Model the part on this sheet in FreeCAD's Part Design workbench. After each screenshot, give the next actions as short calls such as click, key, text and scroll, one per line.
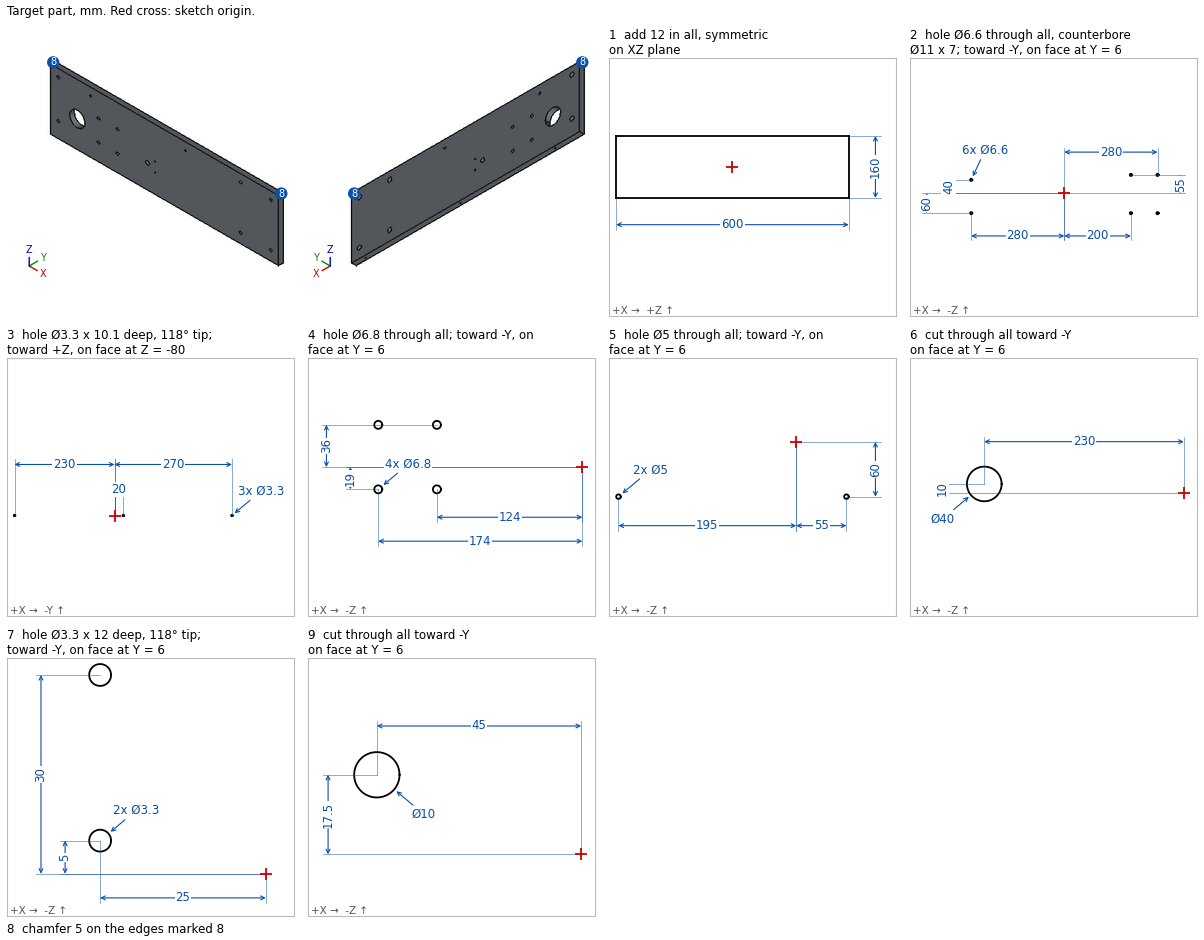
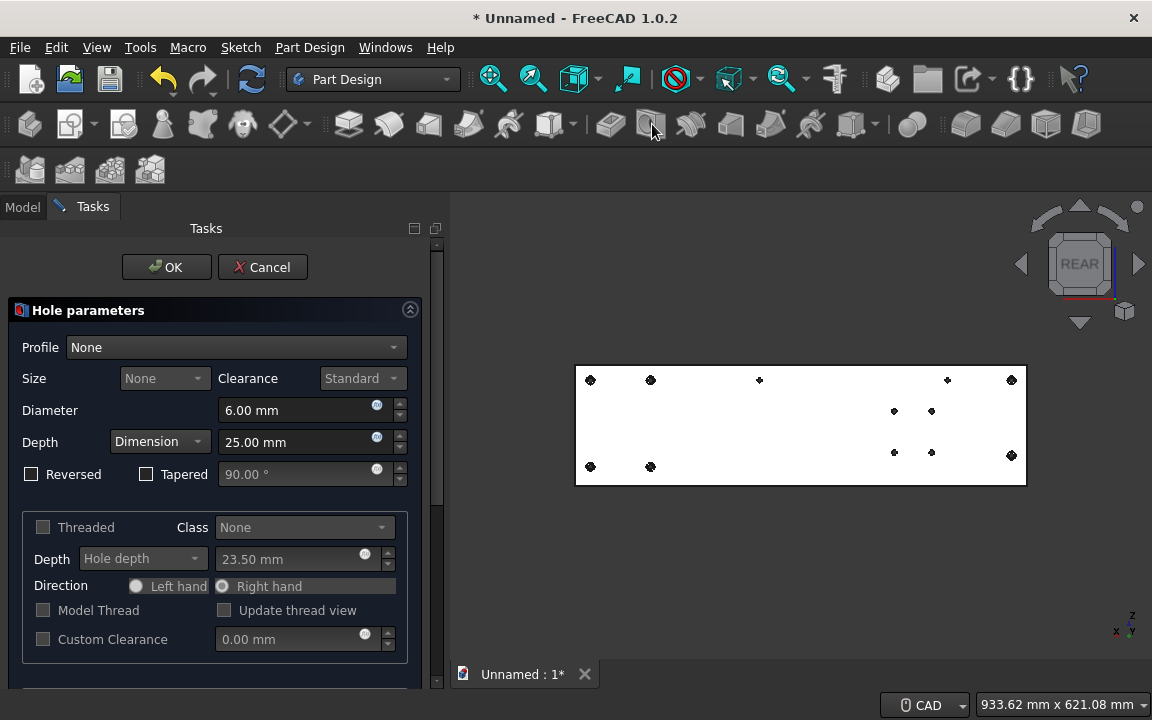
triple_click(305, 410)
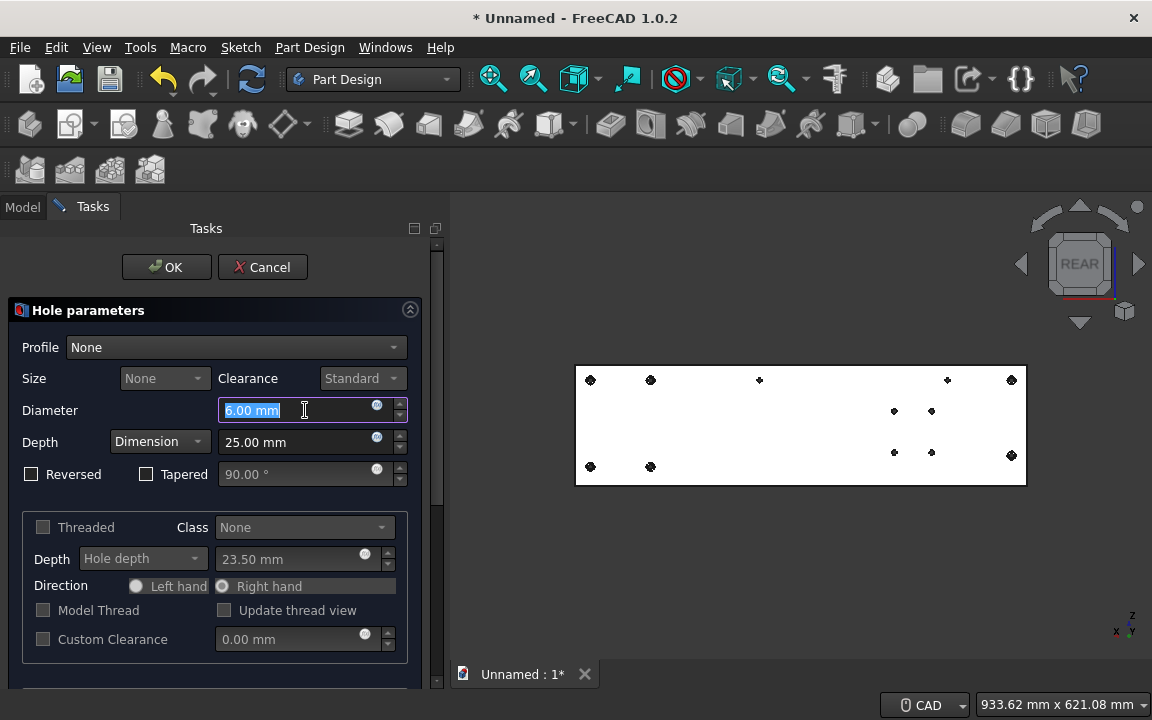
text(5)
key(Tab)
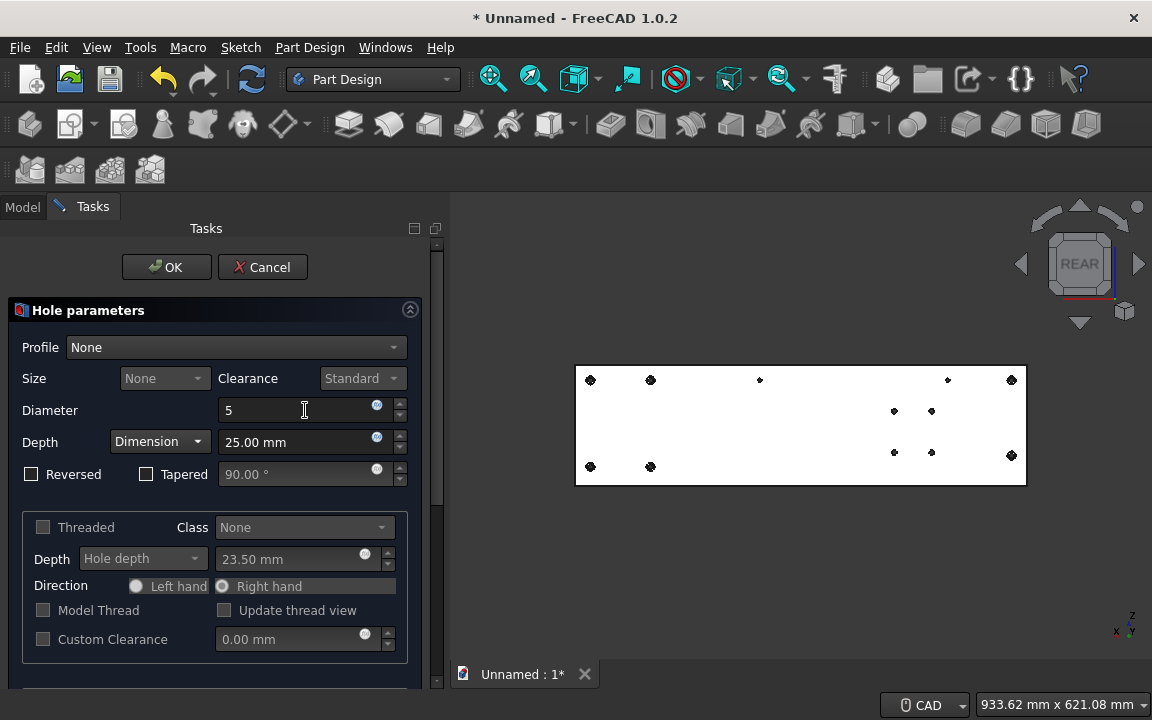
click(161, 442)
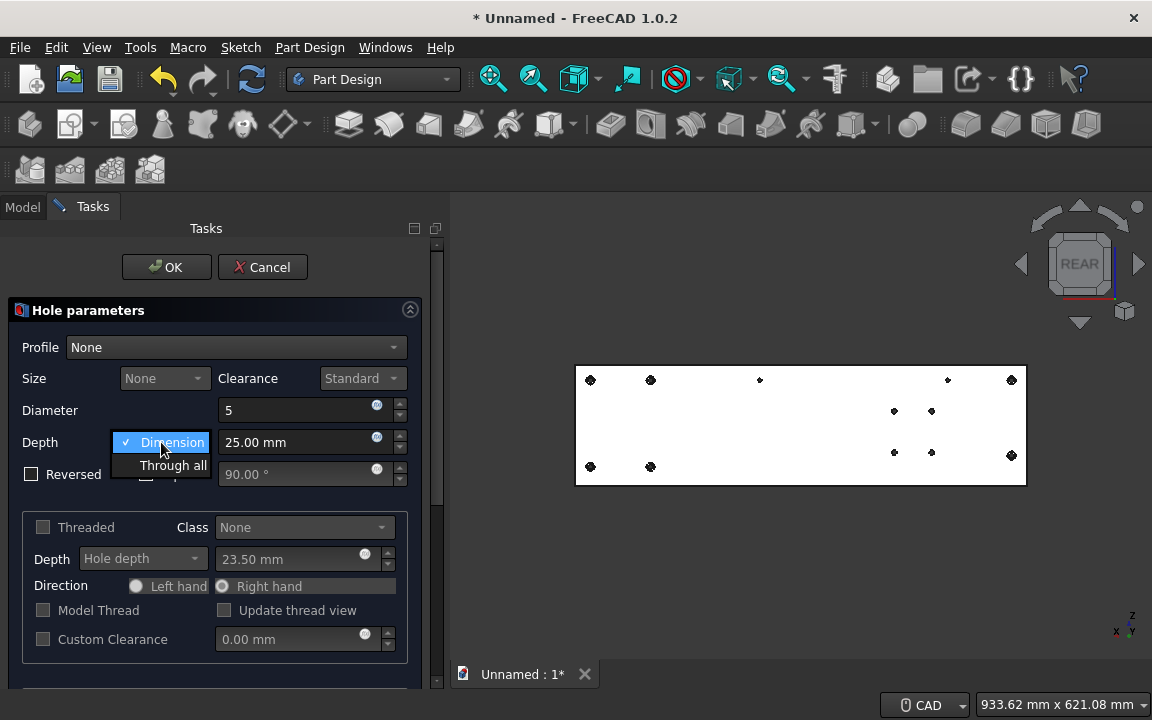
click(160, 466)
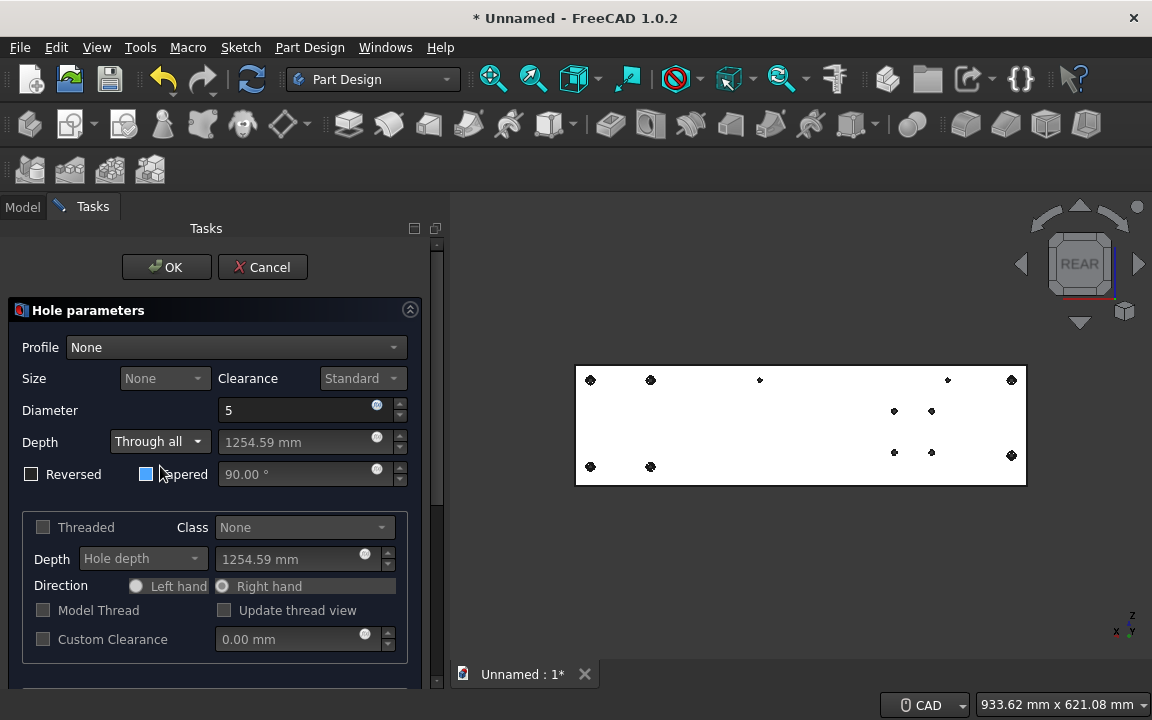
click(167, 267)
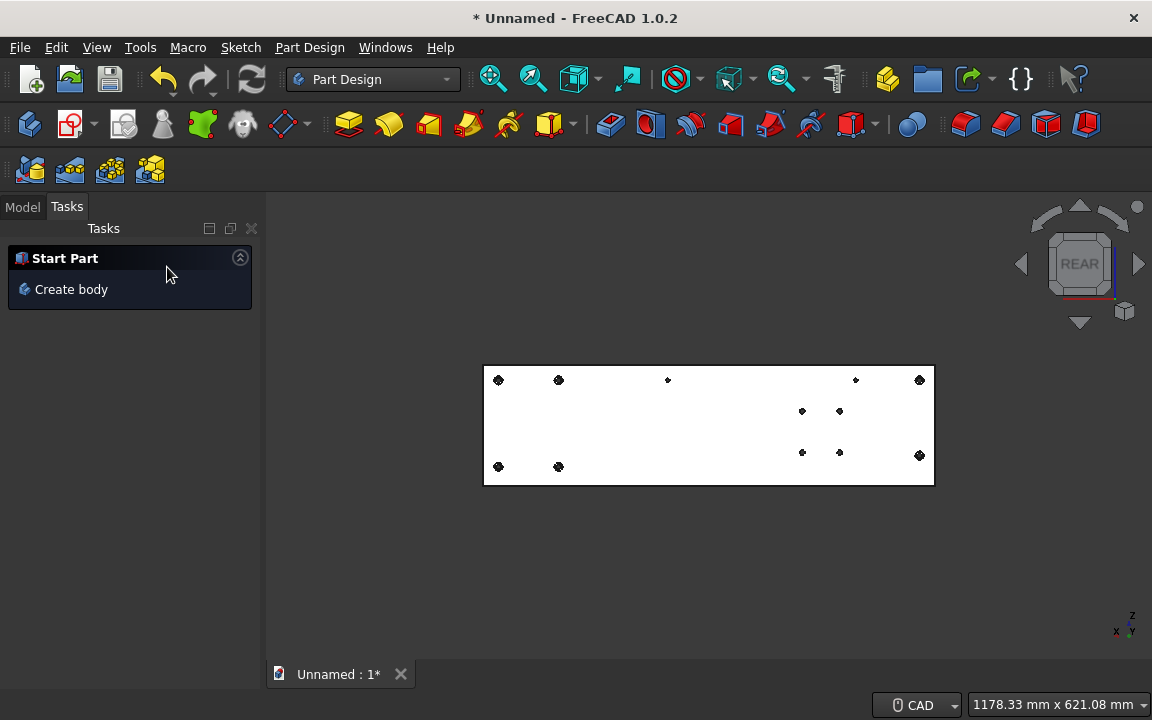
click(709, 424)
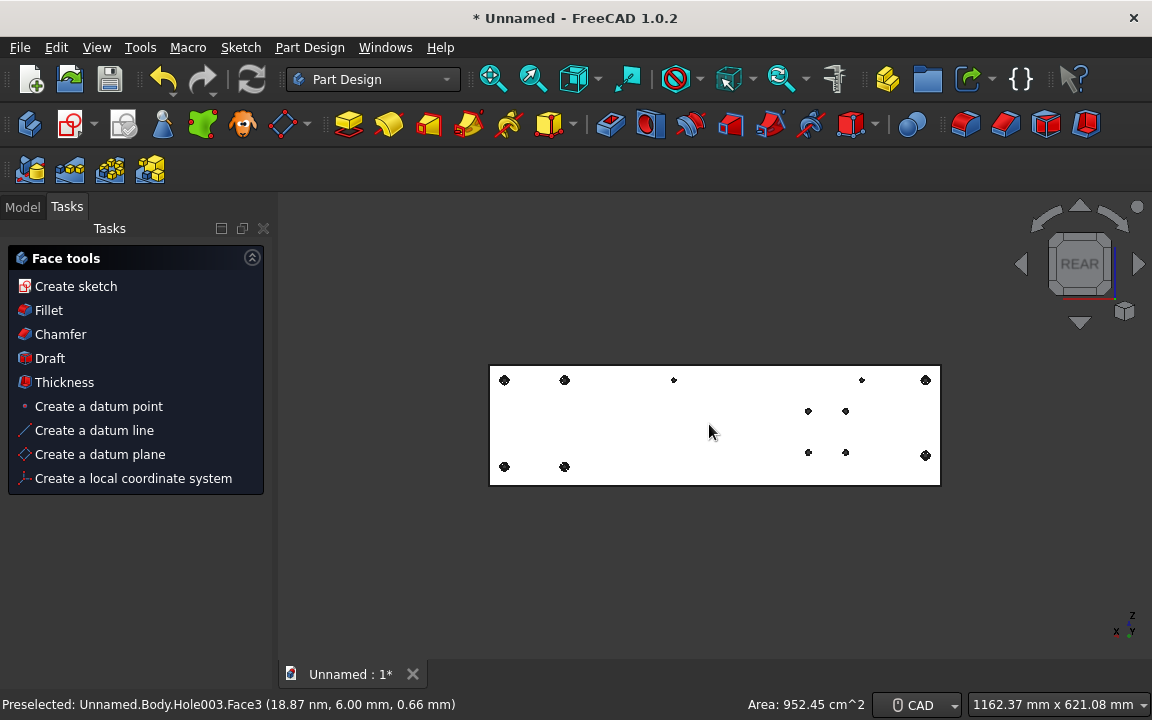
click(70, 124)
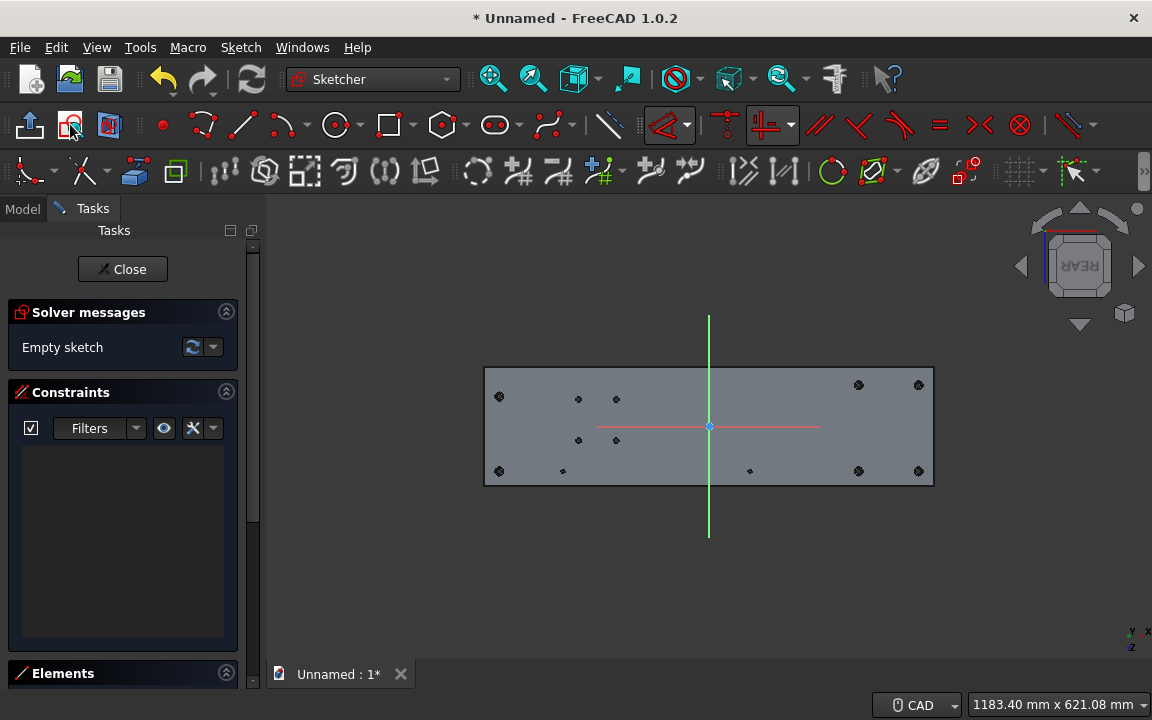
scroll(524, 418, up, 11)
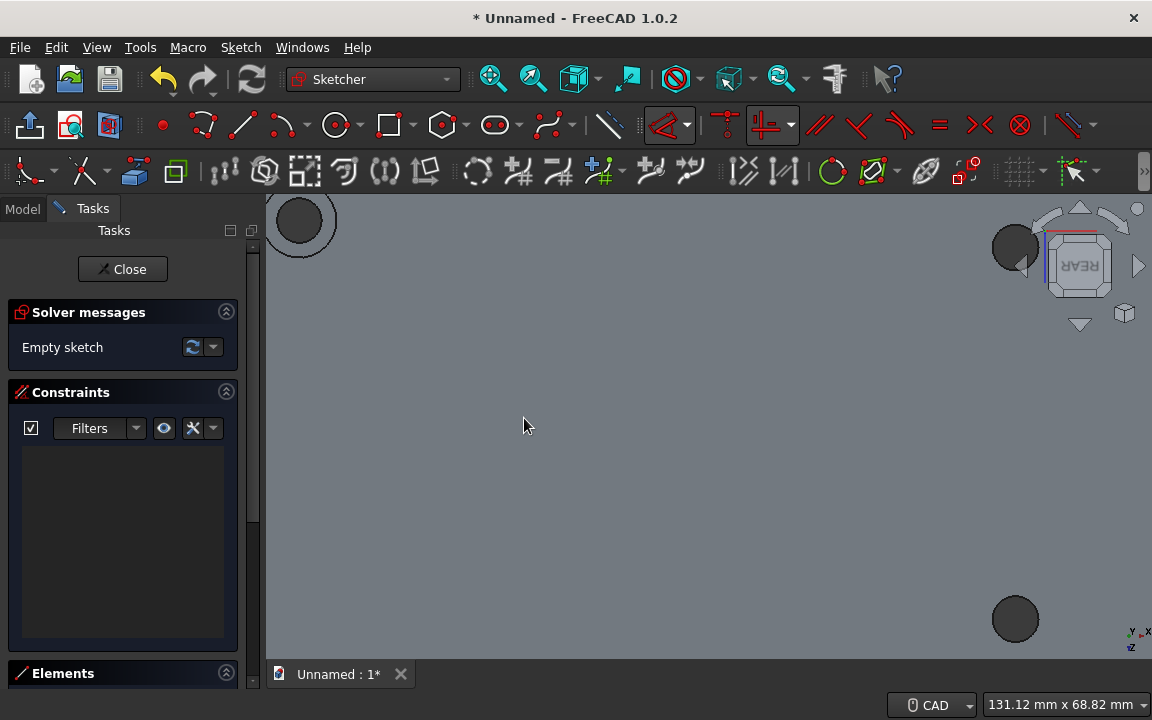
click(336, 126)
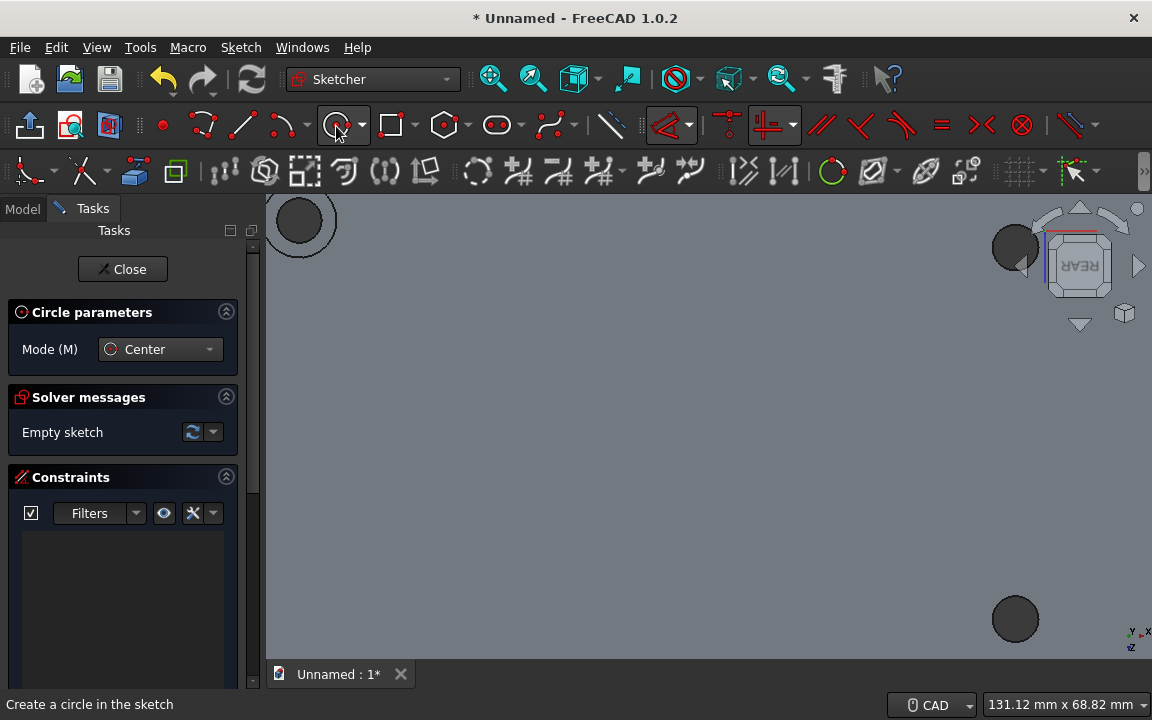
click(637, 423)
move(733, 328)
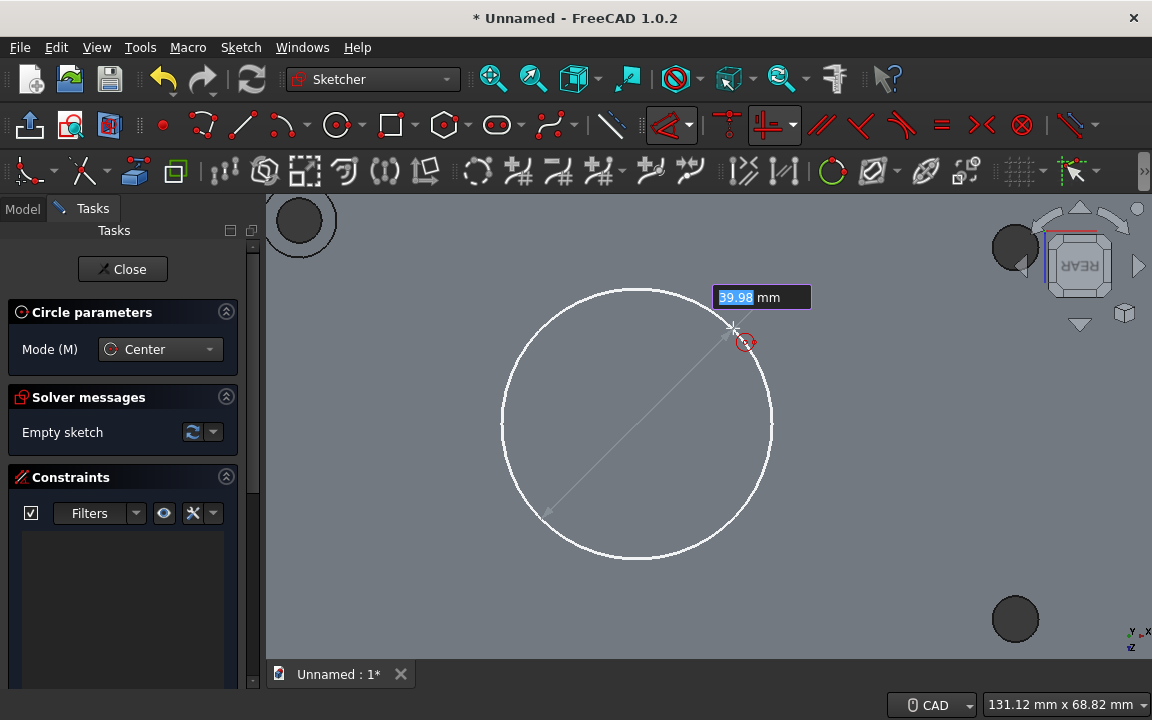
text(40)
key(Return)
key(Escape)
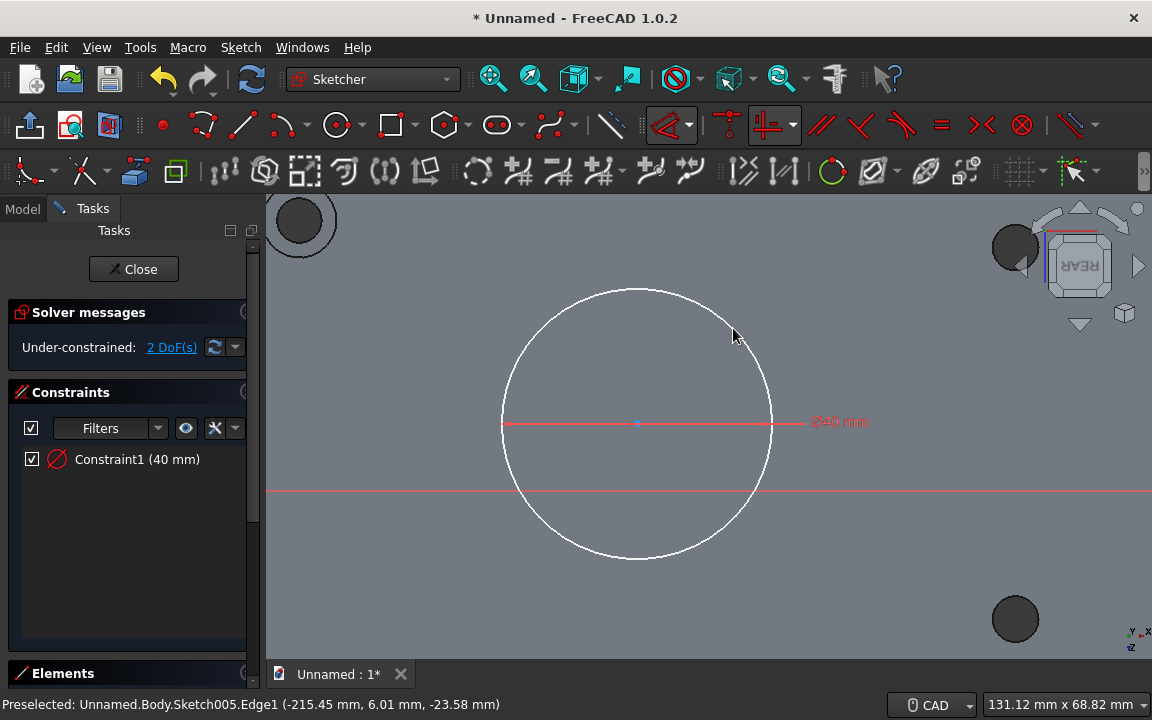
click(637, 424)